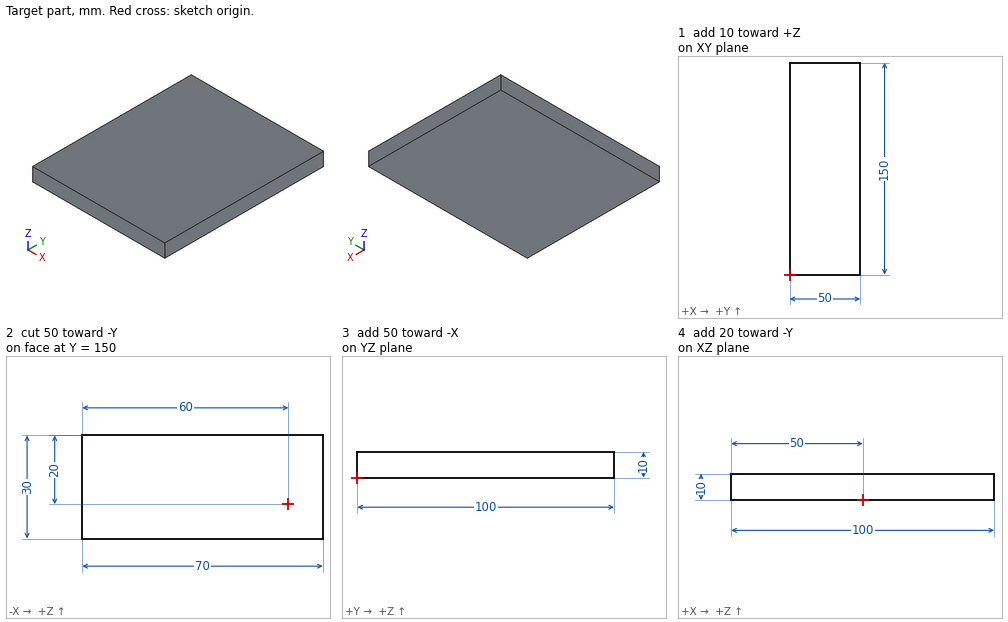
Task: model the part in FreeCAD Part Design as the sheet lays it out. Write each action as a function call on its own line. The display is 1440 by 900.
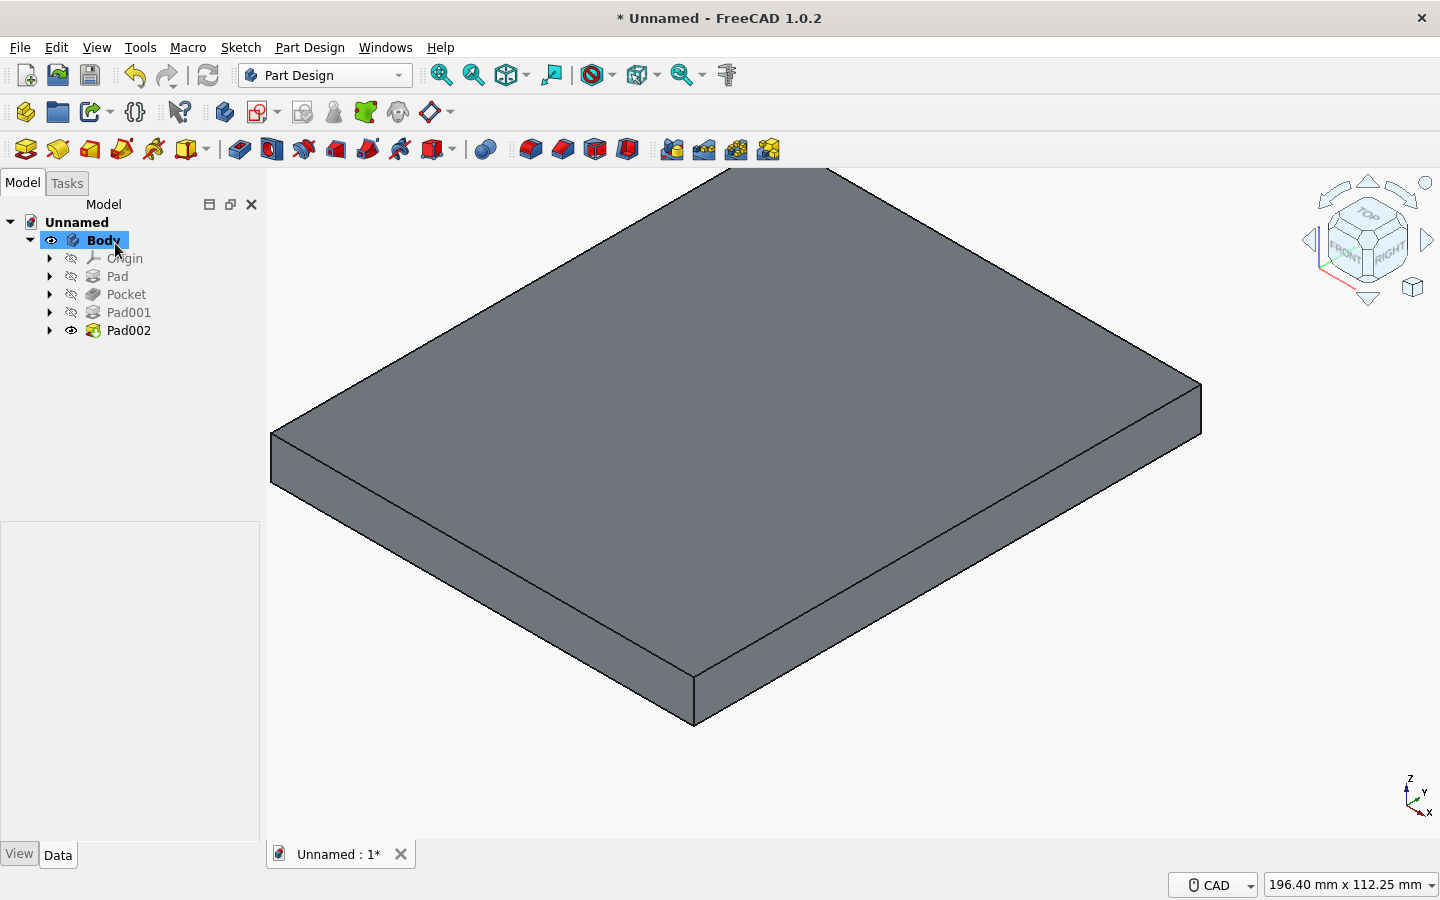
click(442, 76)